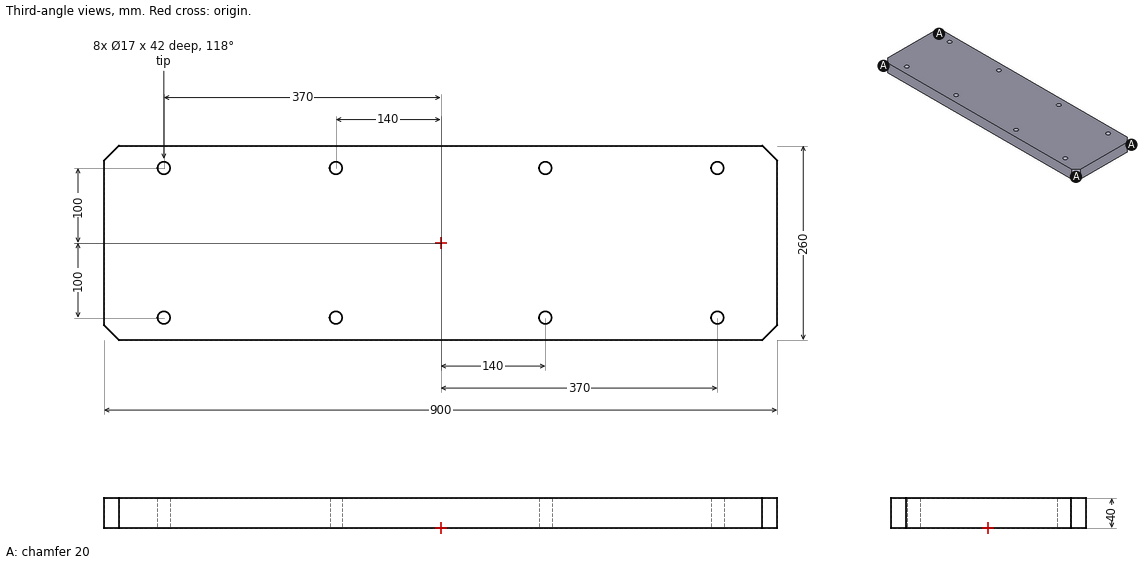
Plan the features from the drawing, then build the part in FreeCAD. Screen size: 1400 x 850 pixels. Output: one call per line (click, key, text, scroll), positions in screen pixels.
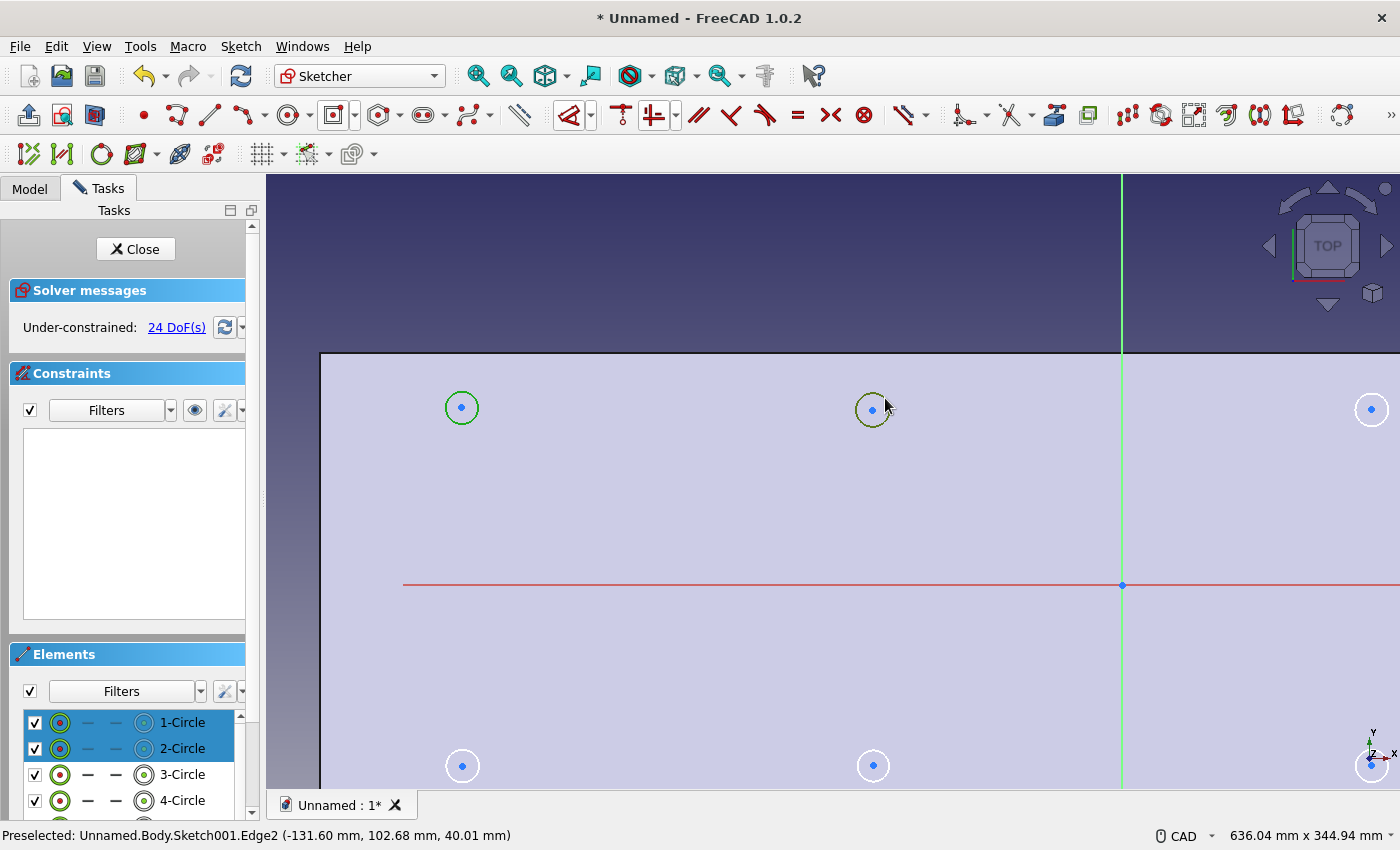
click(474, 755)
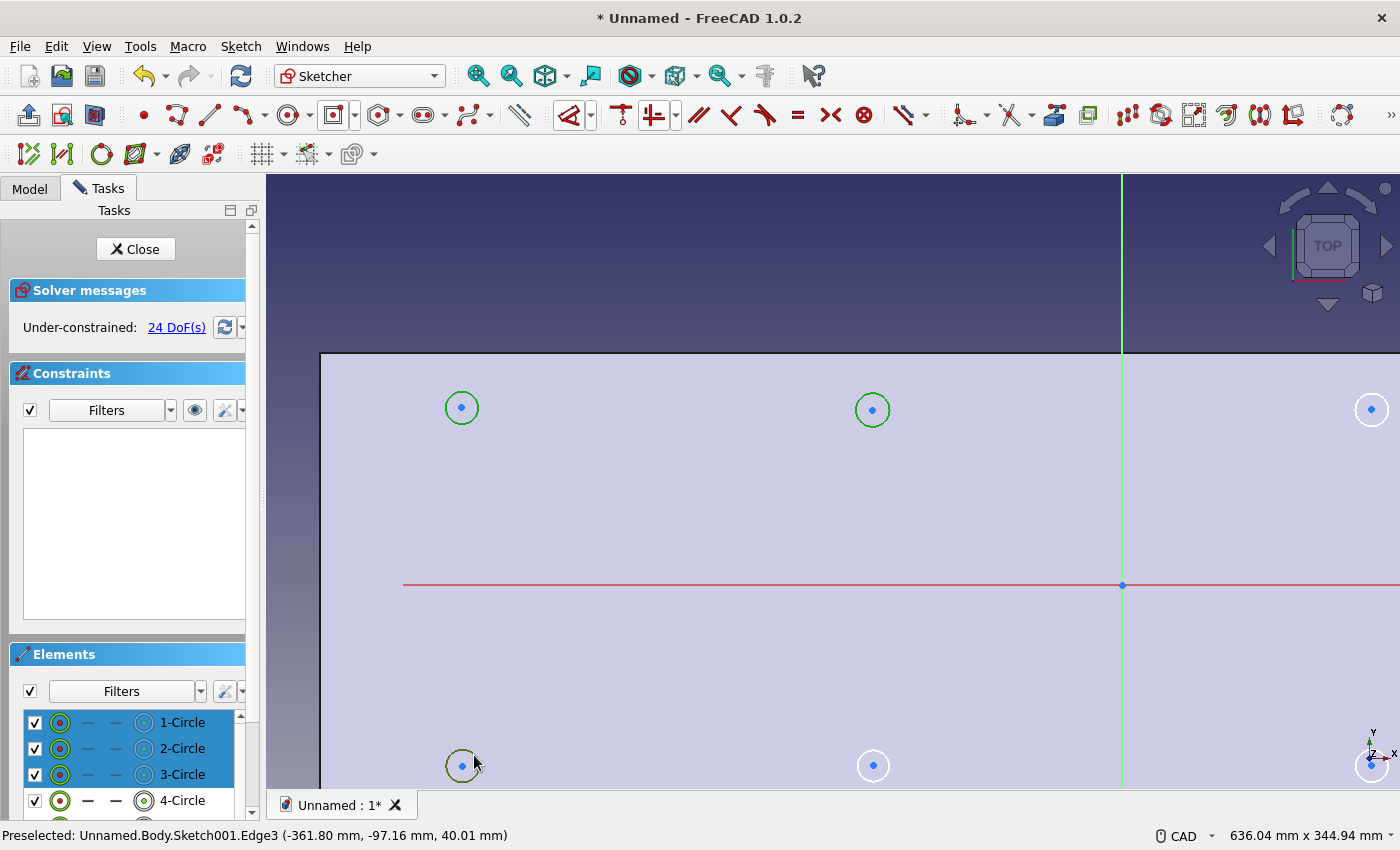
click(884, 755)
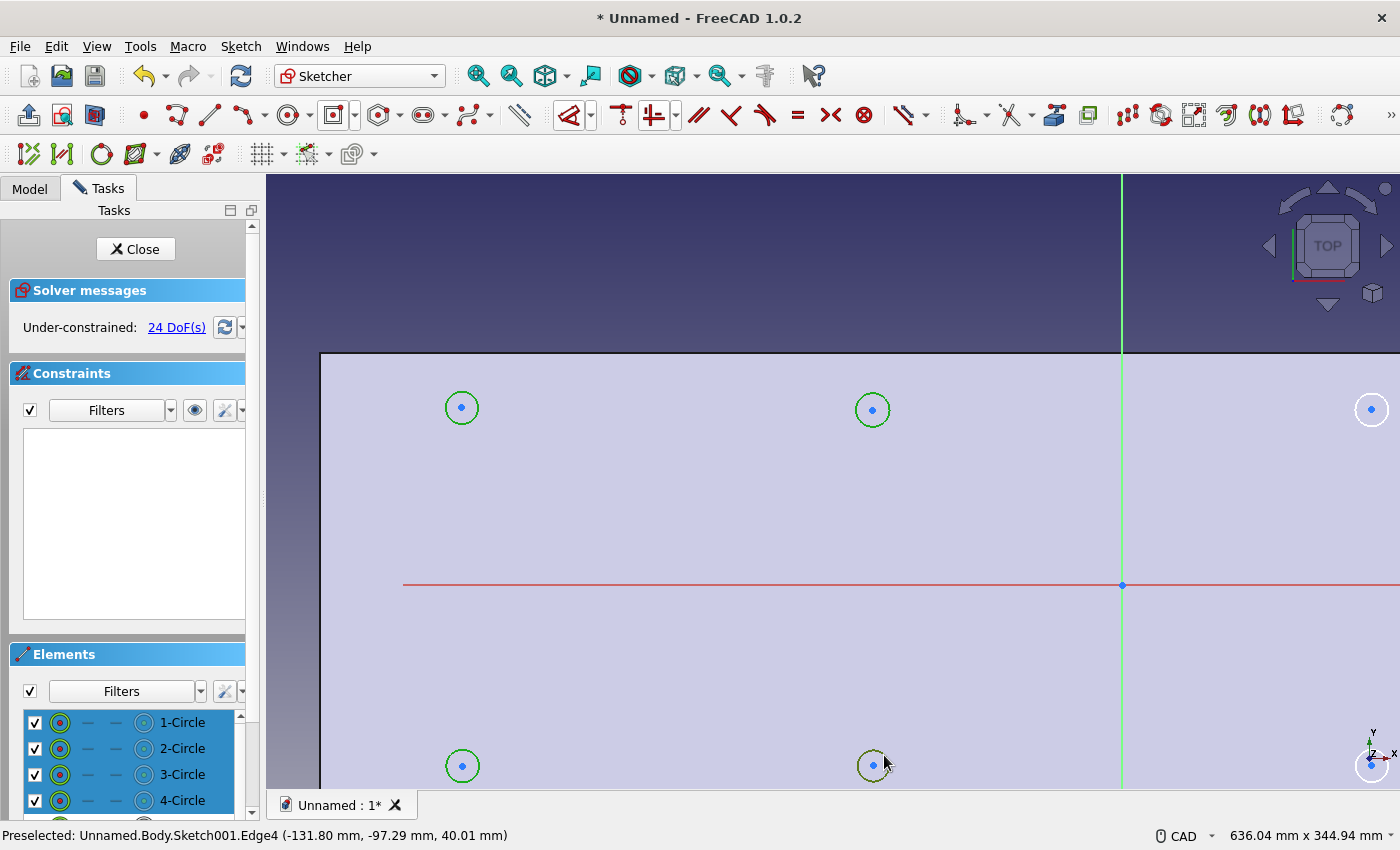
scroll(473, 397, down, 4)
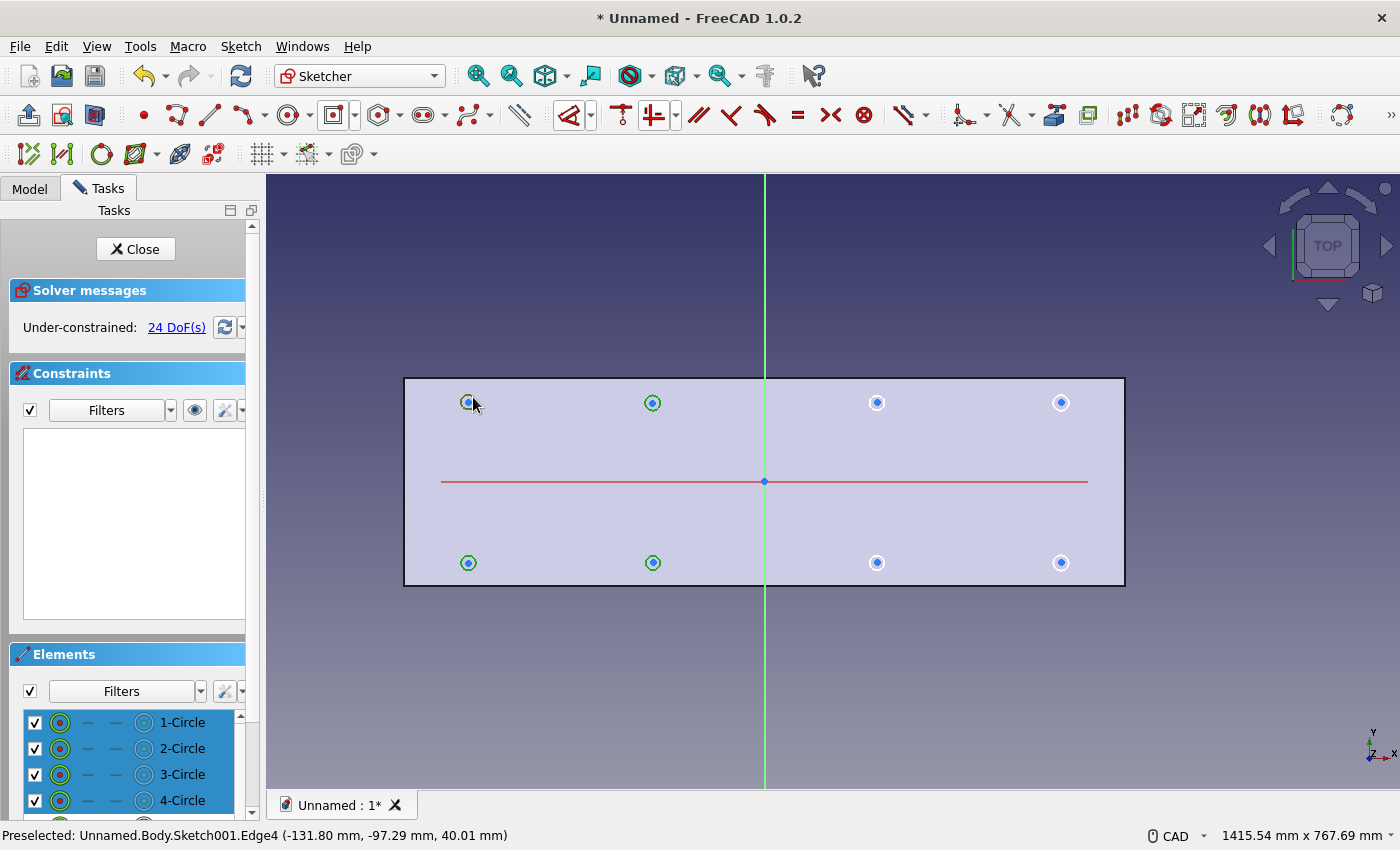
scroll(882, 558, up, 4)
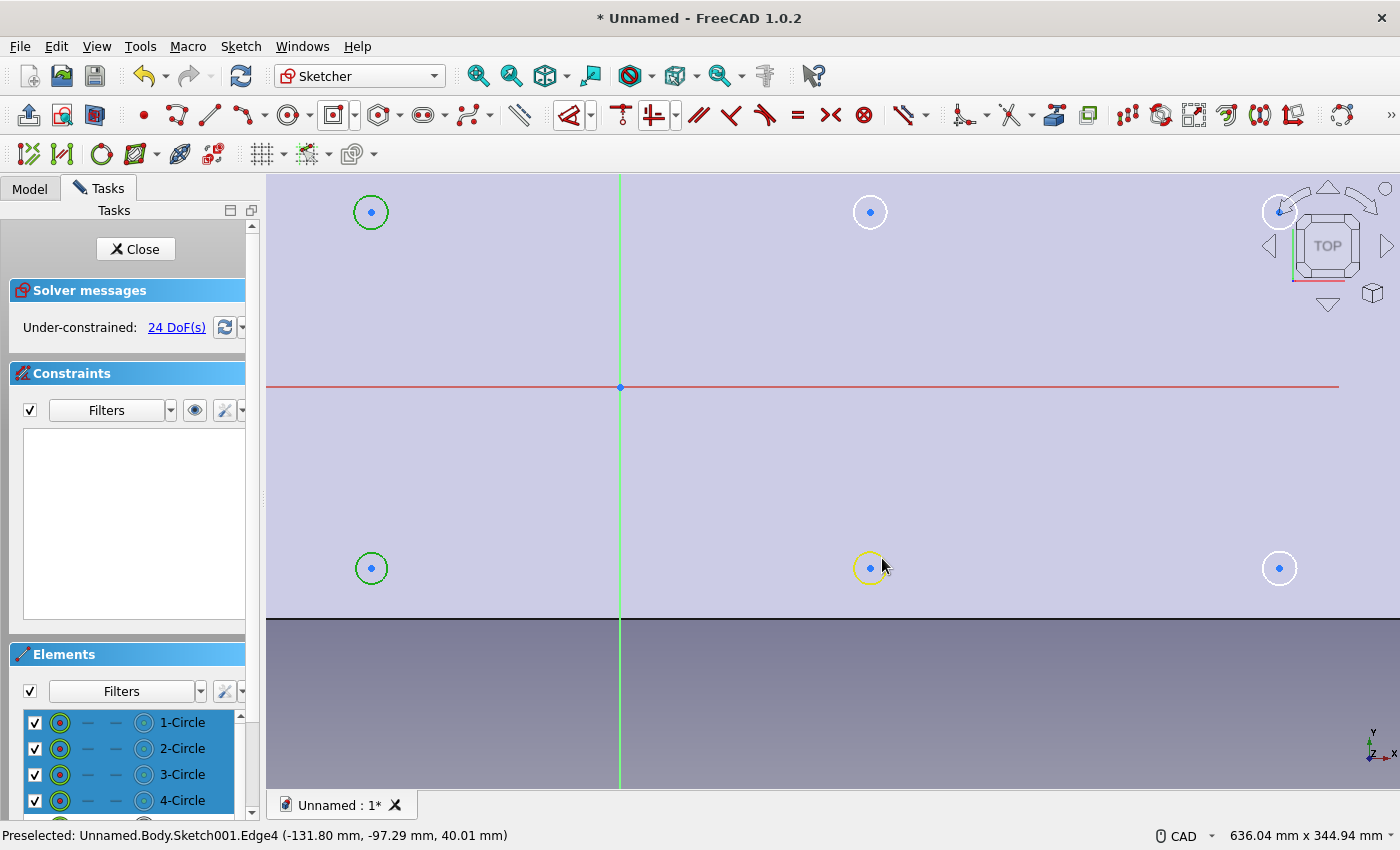
click(882, 557)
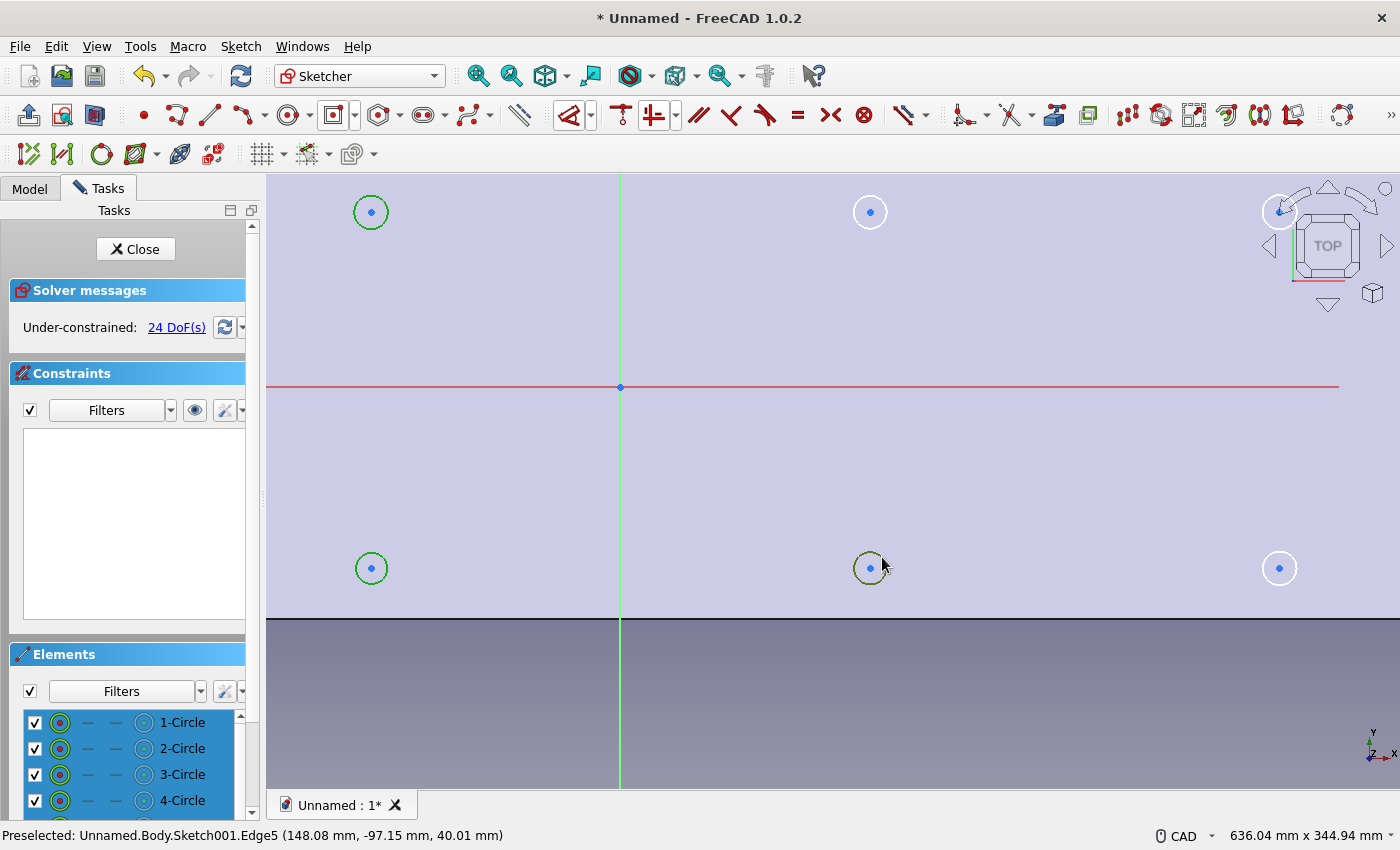
scroll(882, 558, down, 4)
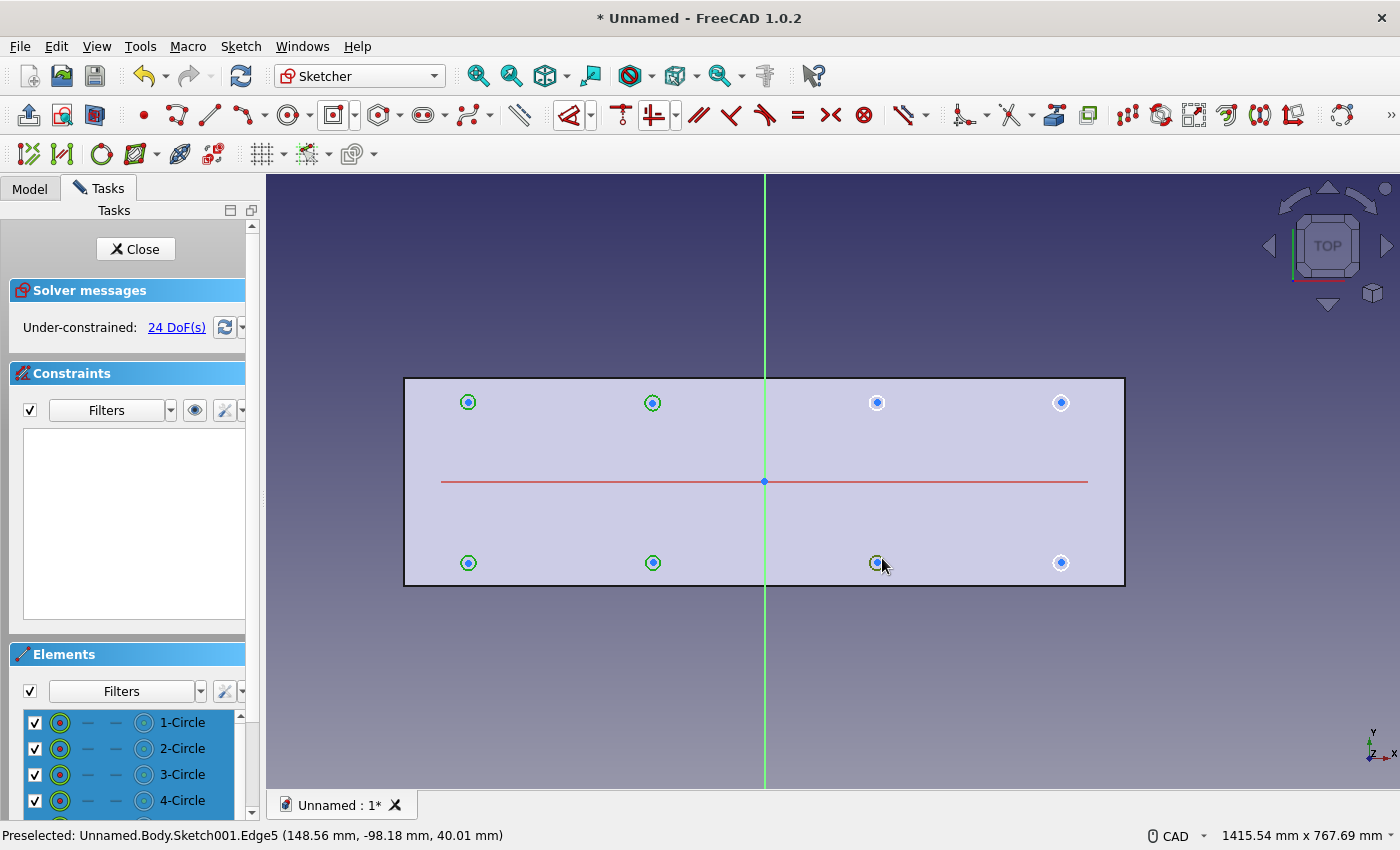
scroll(1066, 558, up, 4)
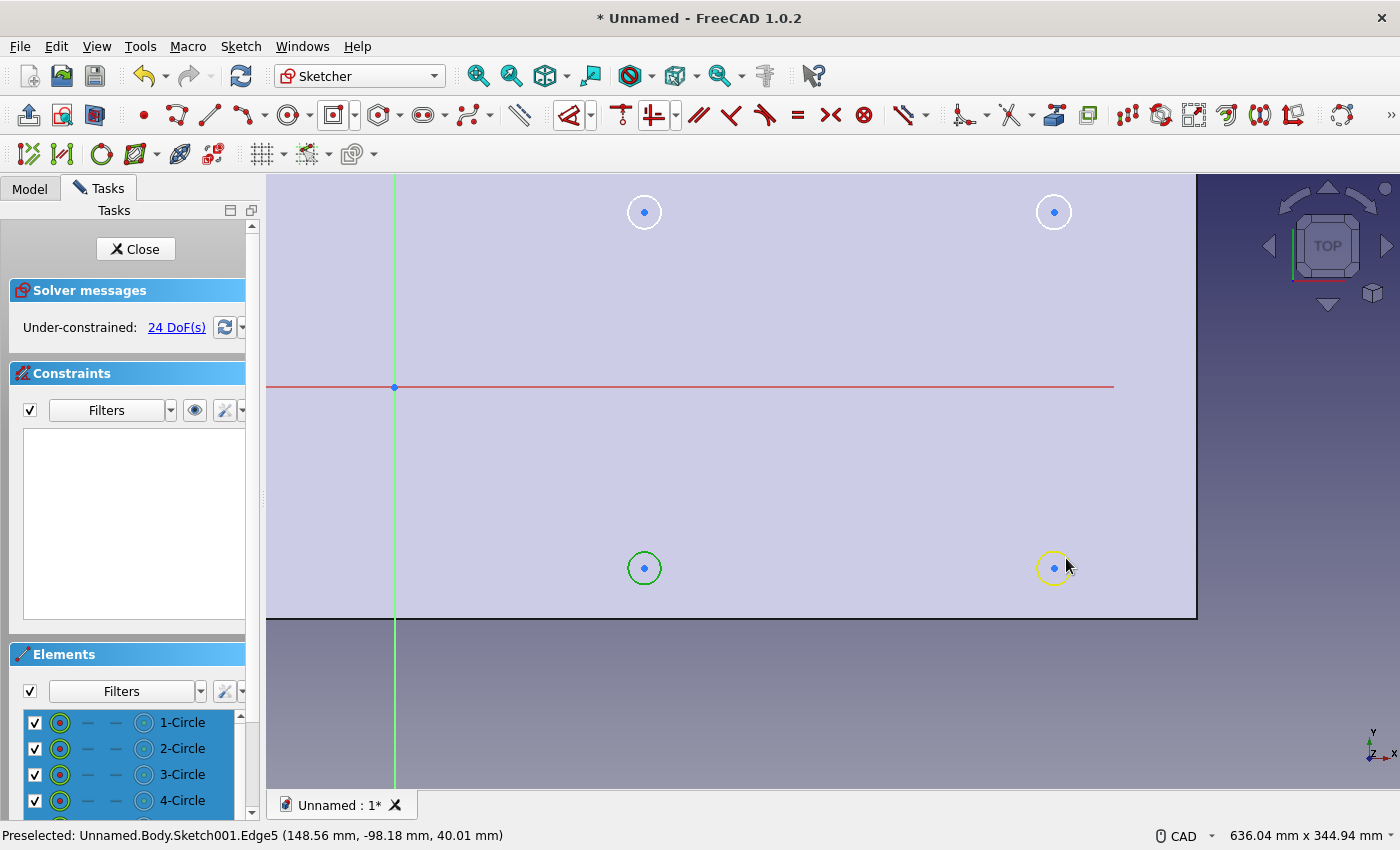
click(1066, 556)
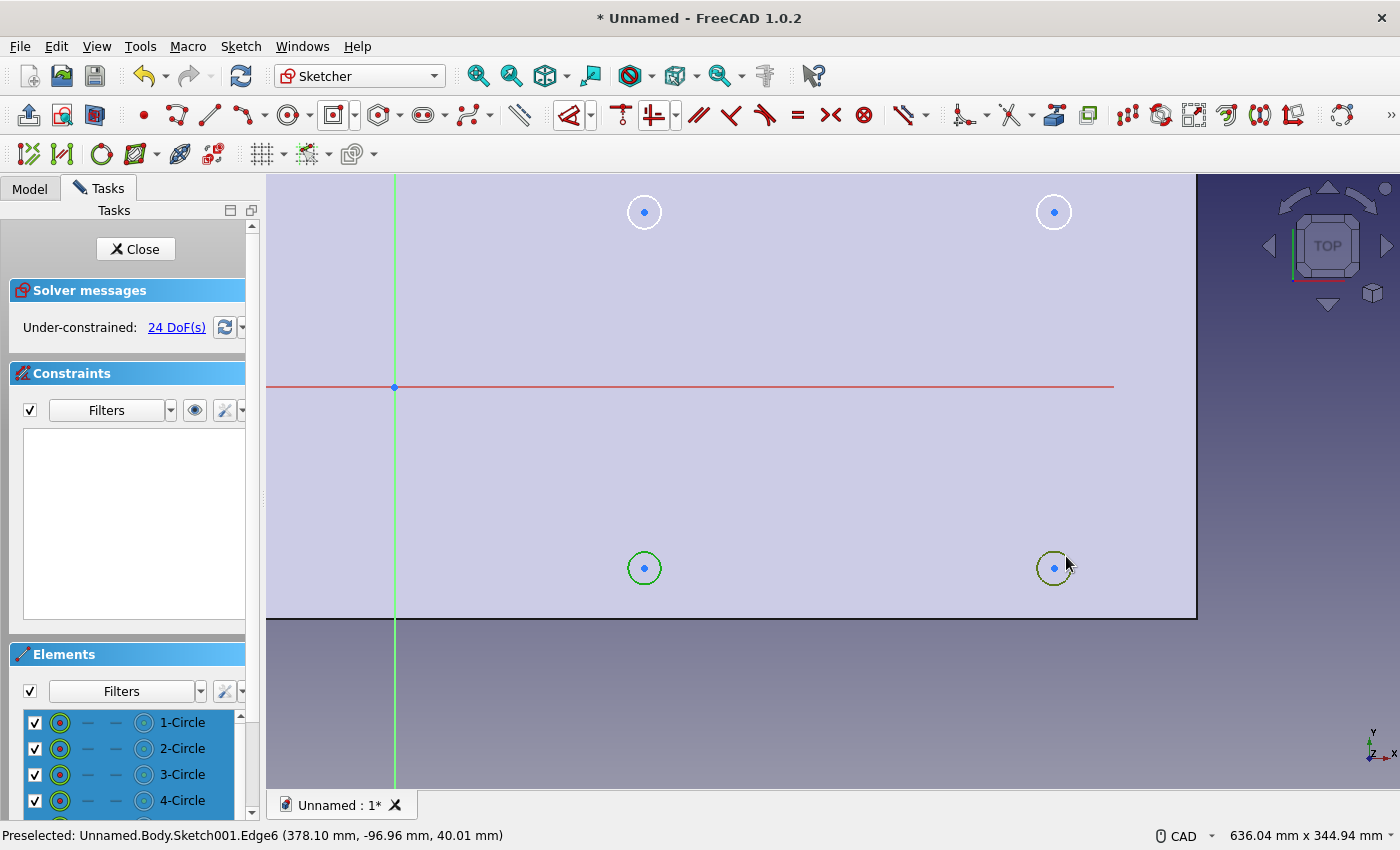
click(633, 224)